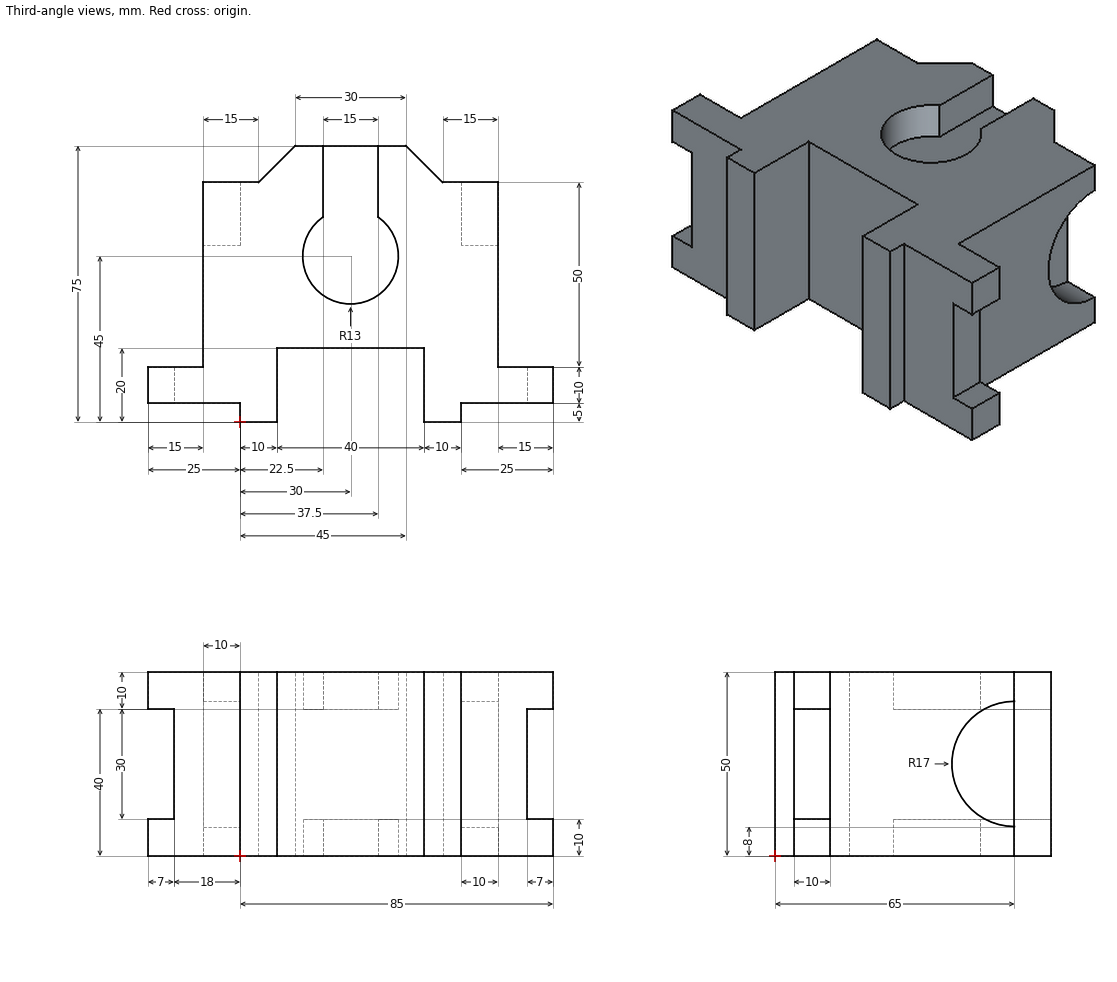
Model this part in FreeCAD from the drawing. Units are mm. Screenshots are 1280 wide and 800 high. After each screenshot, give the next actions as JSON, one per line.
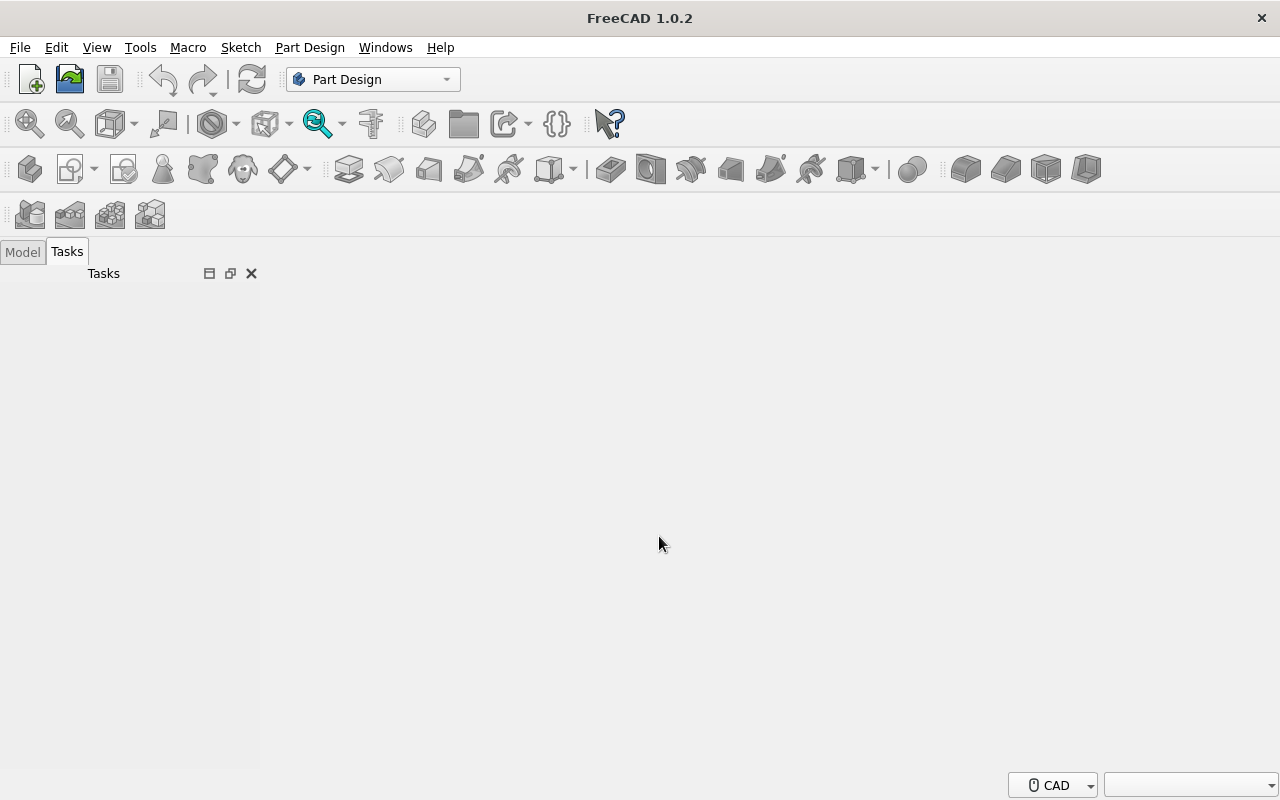
{"action": "left_click", "coordinate": [30, 80]}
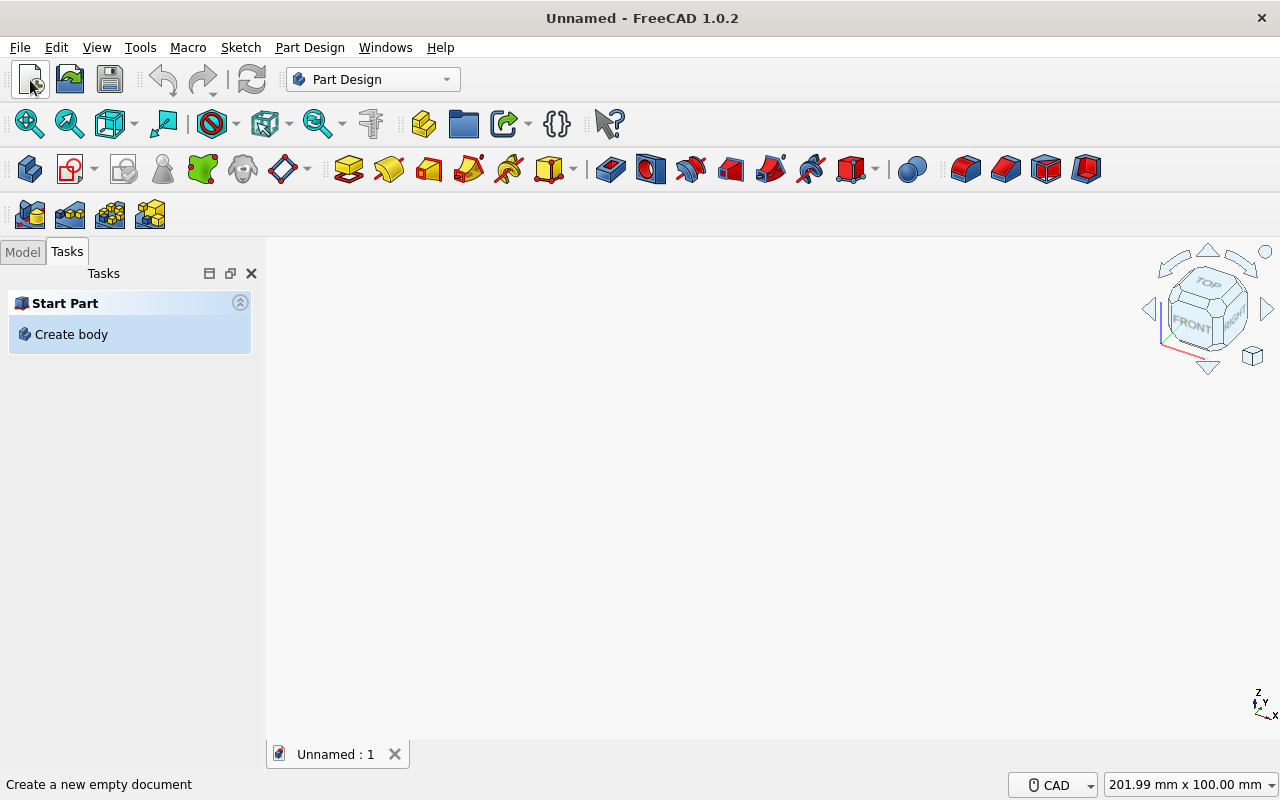
{"action": "left_click", "coordinate": [70, 170]}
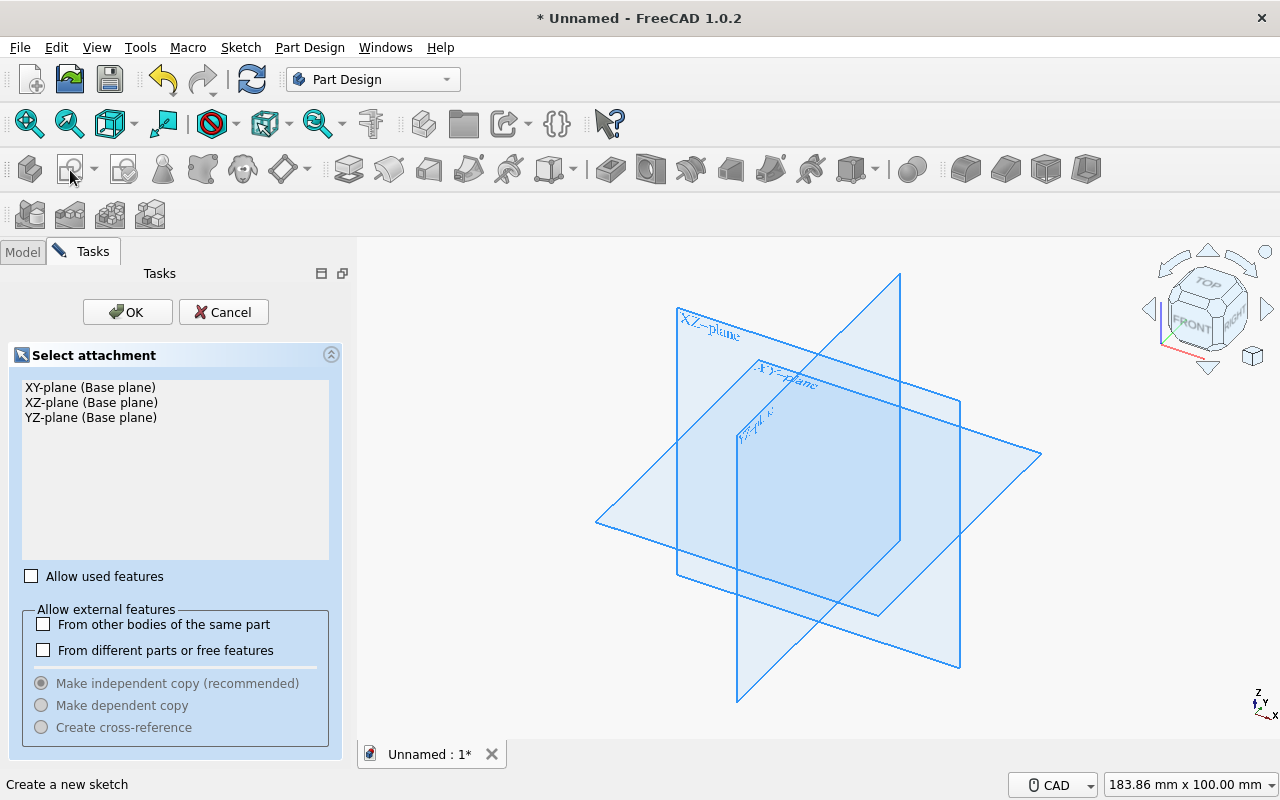
{"action": "left_click", "coordinate": [82, 388]}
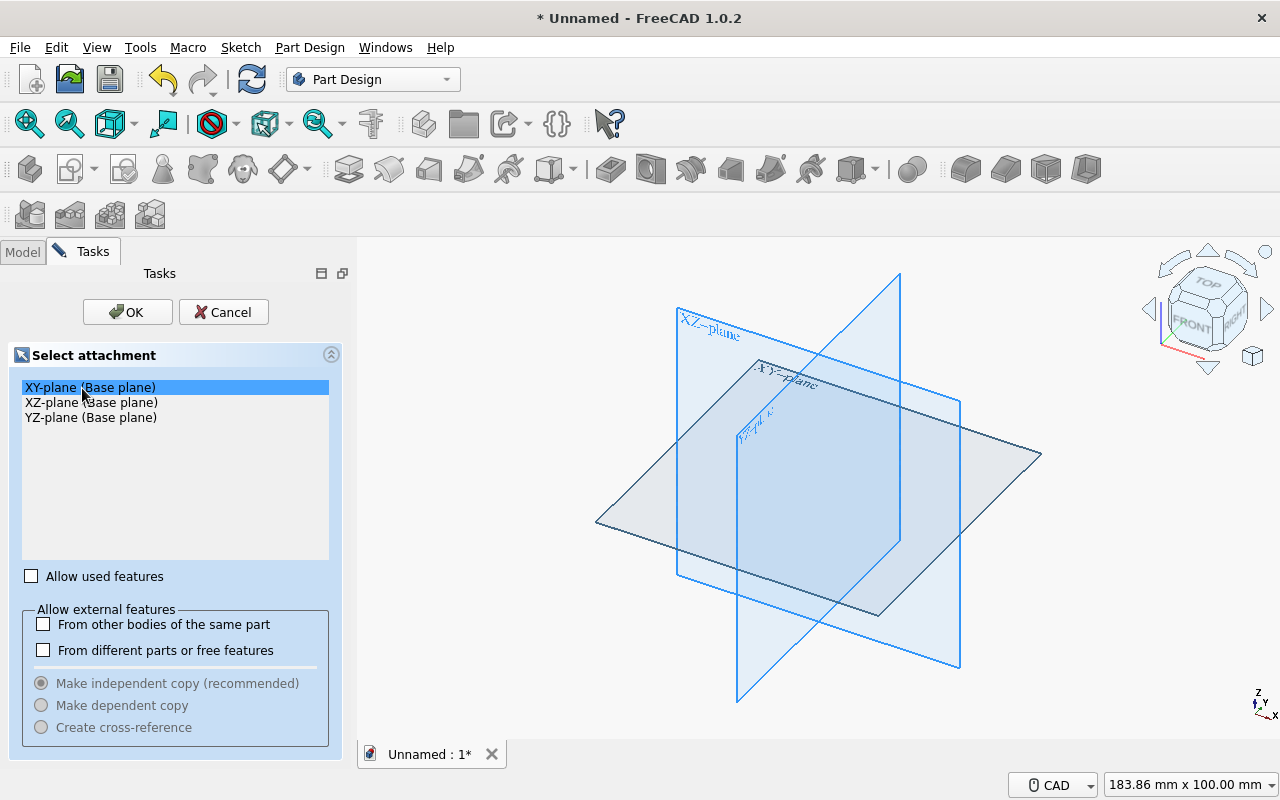
{"action": "left_click", "coordinate": [128, 312]}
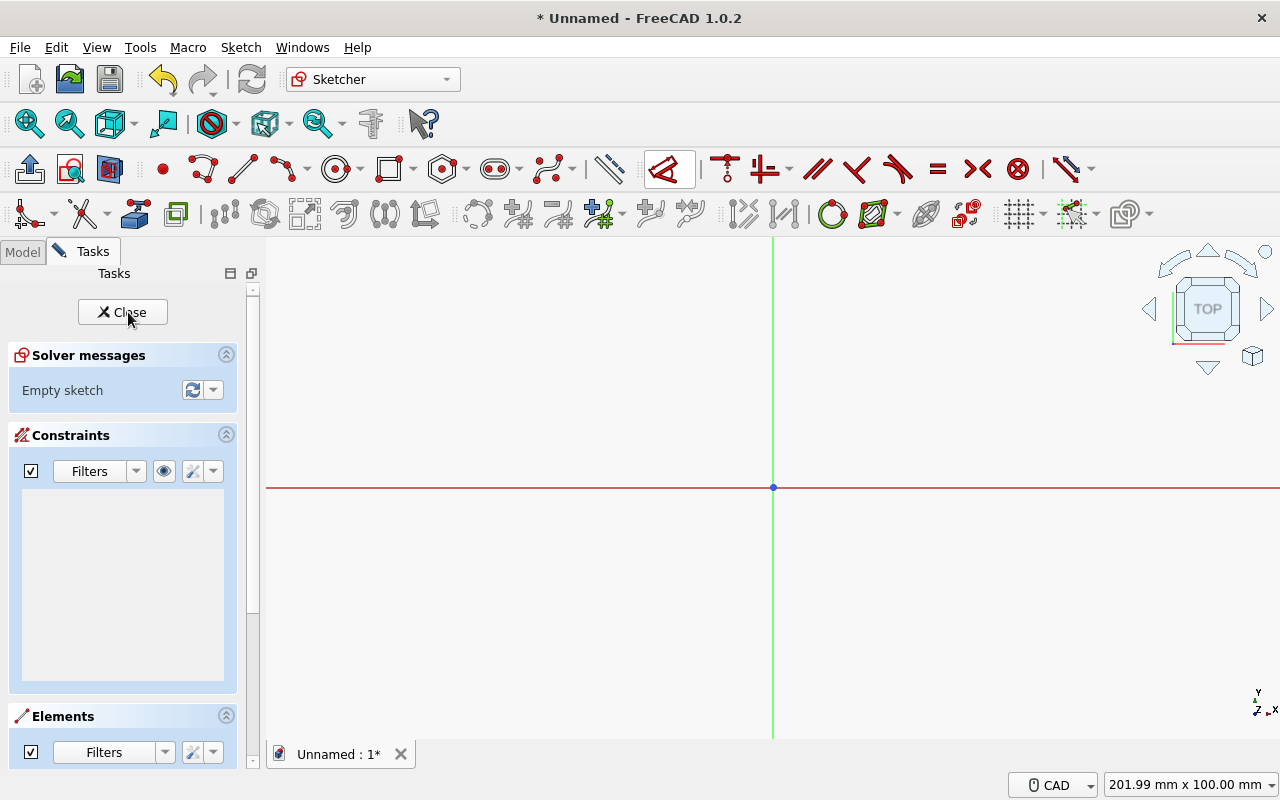
{"action": "scroll", "coordinate": [294, 711], "scroll_direction": "down", "scroll_amount": 2}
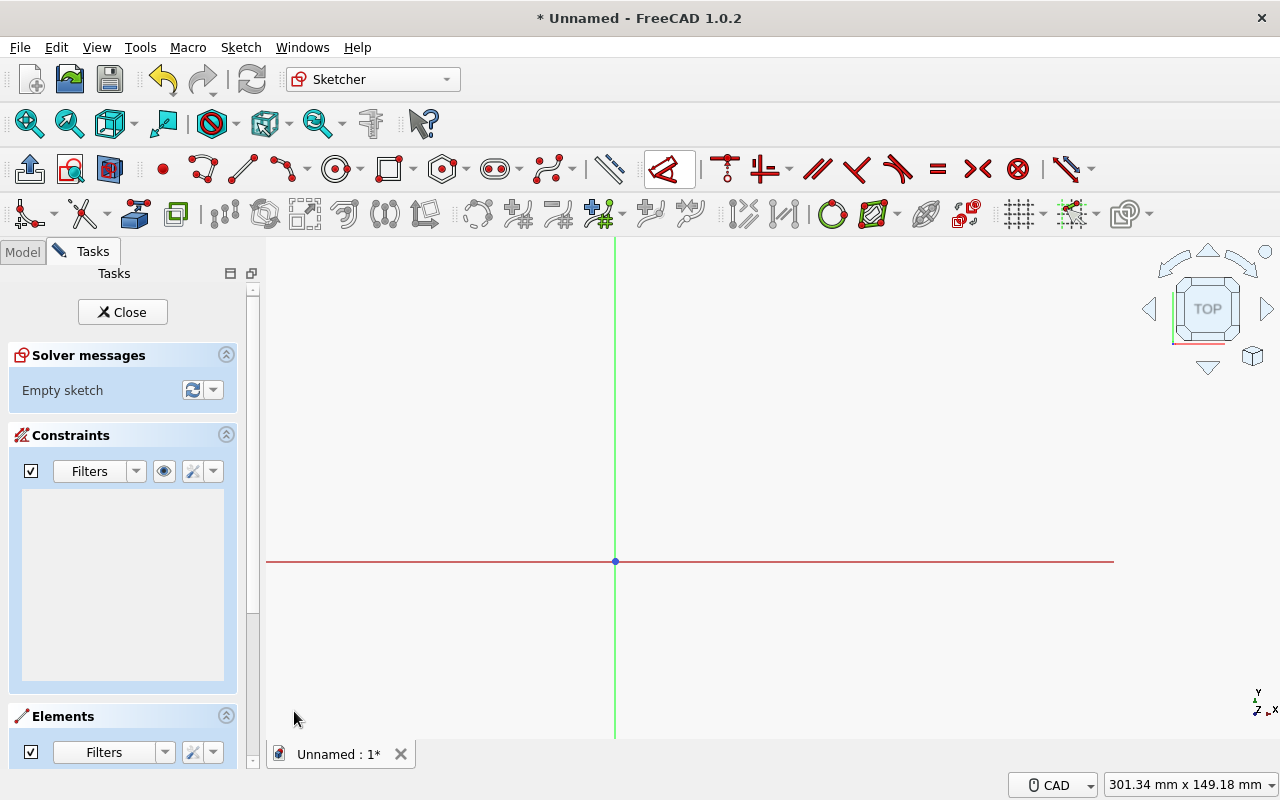
{"action": "left_click", "coordinate": [204, 170]}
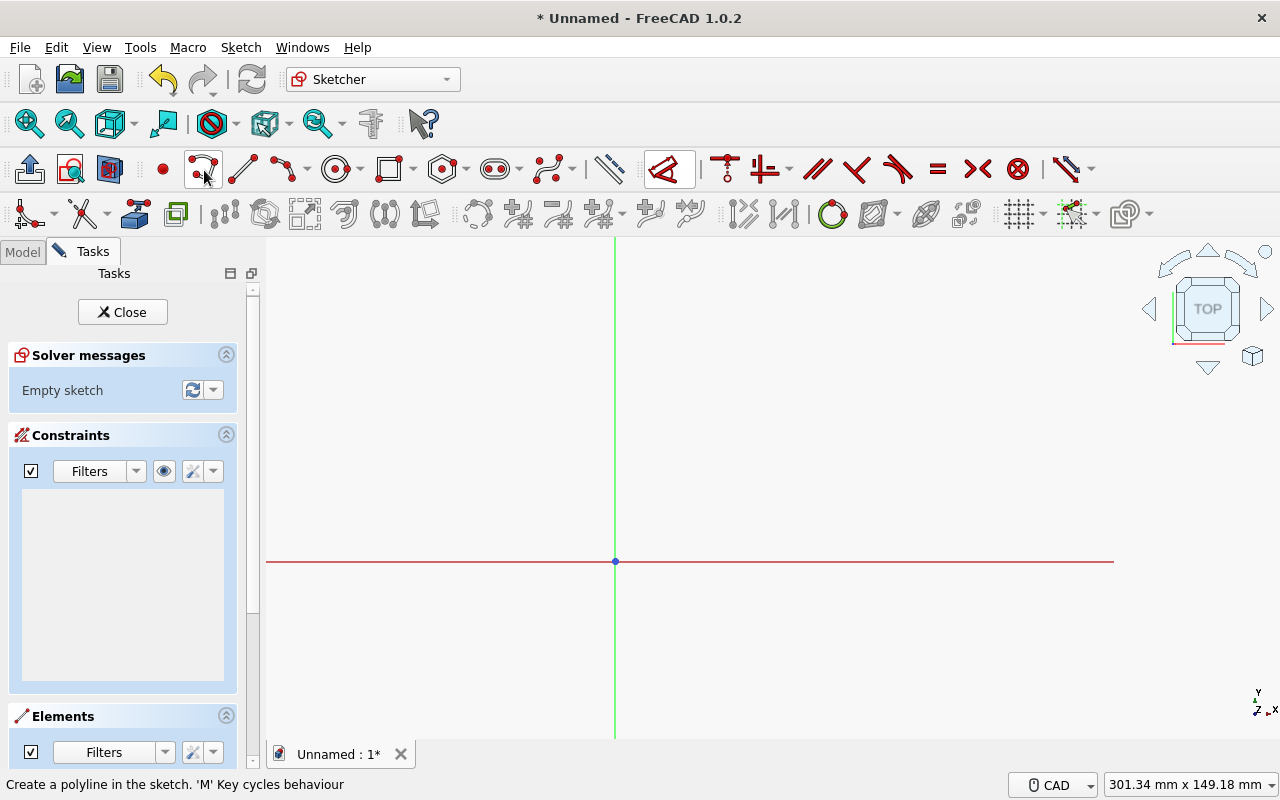
{"action": "left_click", "coordinate": [615, 562]}
{"action": "left_click", "coordinate": [649, 553]}
{"action": "left_click", "coordinate": [649, 495]}
{"action": "left_click", "coordinate": [783, 495]}
{"action": "left_click", "coordinate": [783, 562]}
{"action": "left_click", "coordinate": [817, 553]}
{"action": "left_click", "coordinate": [817, 545]}
{"action": "left_click", "coordinate": [901, 545]}
{"action": "left_click", "coordinate": [901, 511]}
{"action": "left_click", "coordinate": [851, 511]}
{"action": "left_click", "coordinate": [851, 343]}
{"action": "left_click", "coordinate": [800, 343]}
{"action": "left_click", "coordinate": [767, 309]}
{"action": "left_click", "coordinate": [666, 309]}
{"action": "left_click", "coordinate": [632, 343]}
{"action": "left_click", "coordinate": [581, 343]}
{"action": "left_click", "coordinate": [581, 511]}
{"action": "left_click", "coordinate": [531, 511]}
{"action": "left_click", "coordinate": [531, 545]}
{"action": "left_click", "coordinate": [624, 545]}
{"action": "left_click", "coordinate": [615, 562]}
{"action": "key", "text": "Escape"}
{"action": "key", "text": "Escape"}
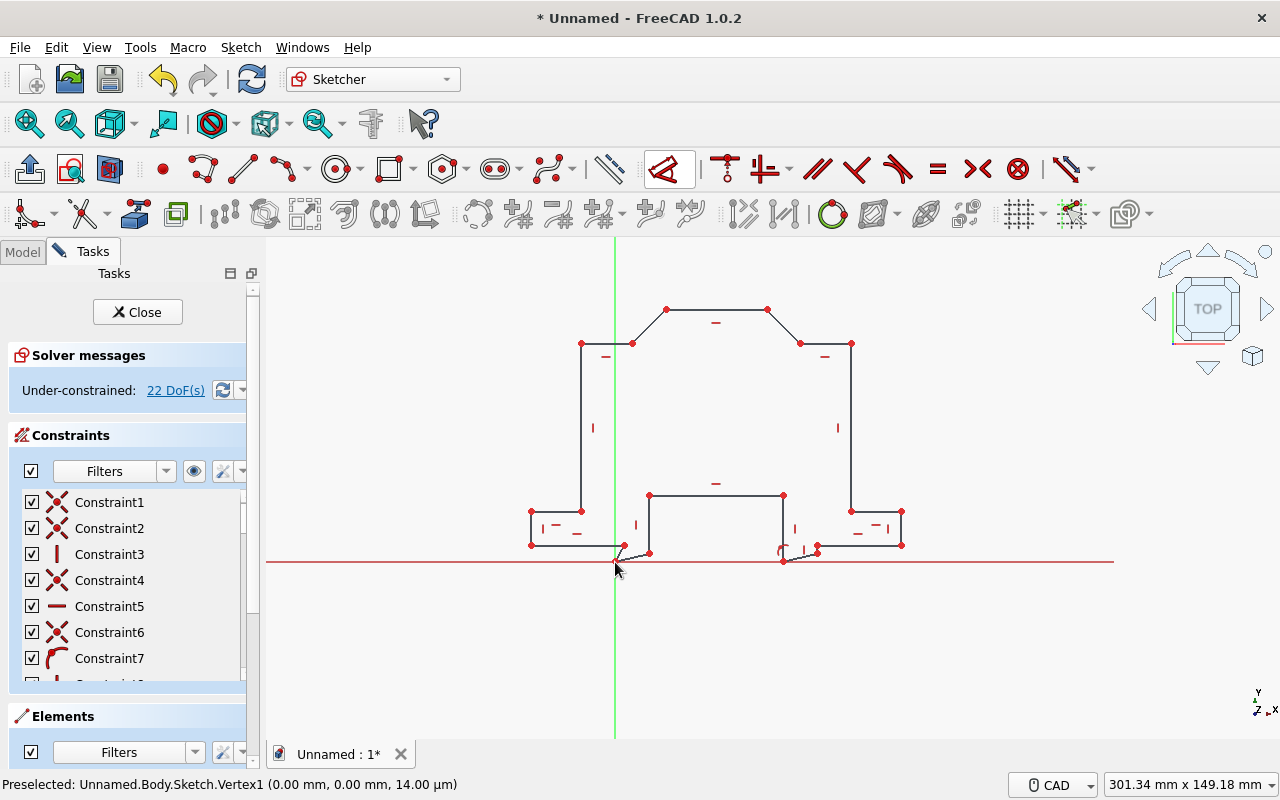
{"action": "scroll", "coordinate": [629, 559], "scroll_direction": "up", "scroll_amount": 2}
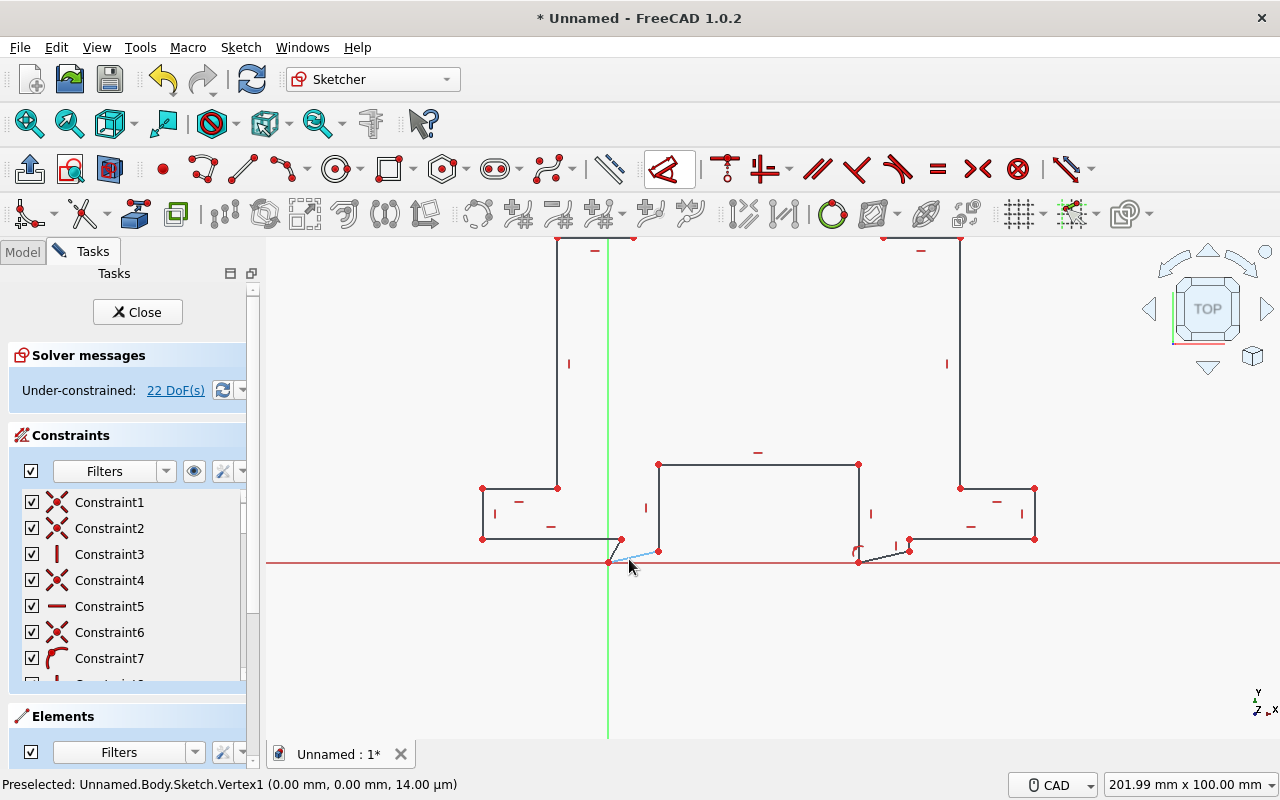
{"action": "left_click", "coordinate": [628, 558]}